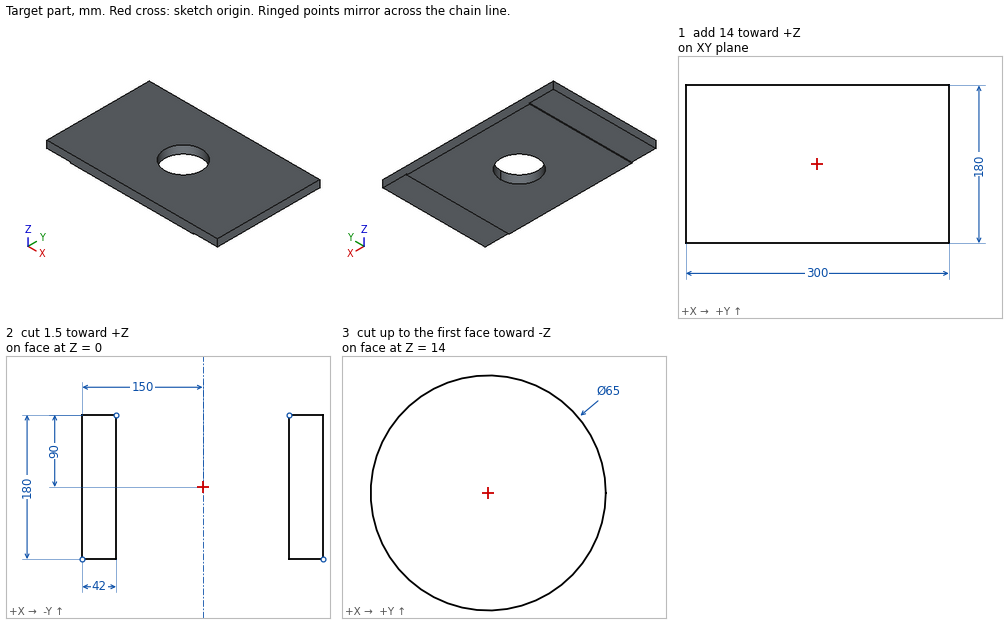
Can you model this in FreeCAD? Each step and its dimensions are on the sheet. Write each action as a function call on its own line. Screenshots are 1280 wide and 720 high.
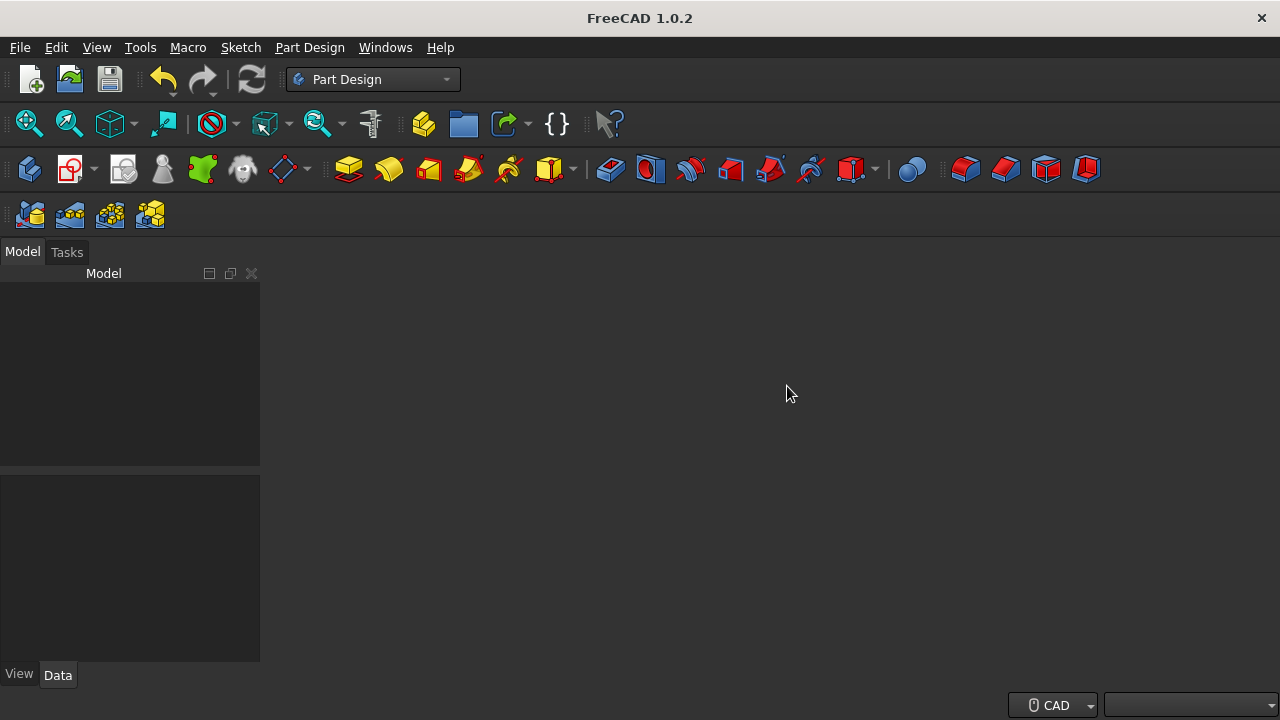
click(30, 80)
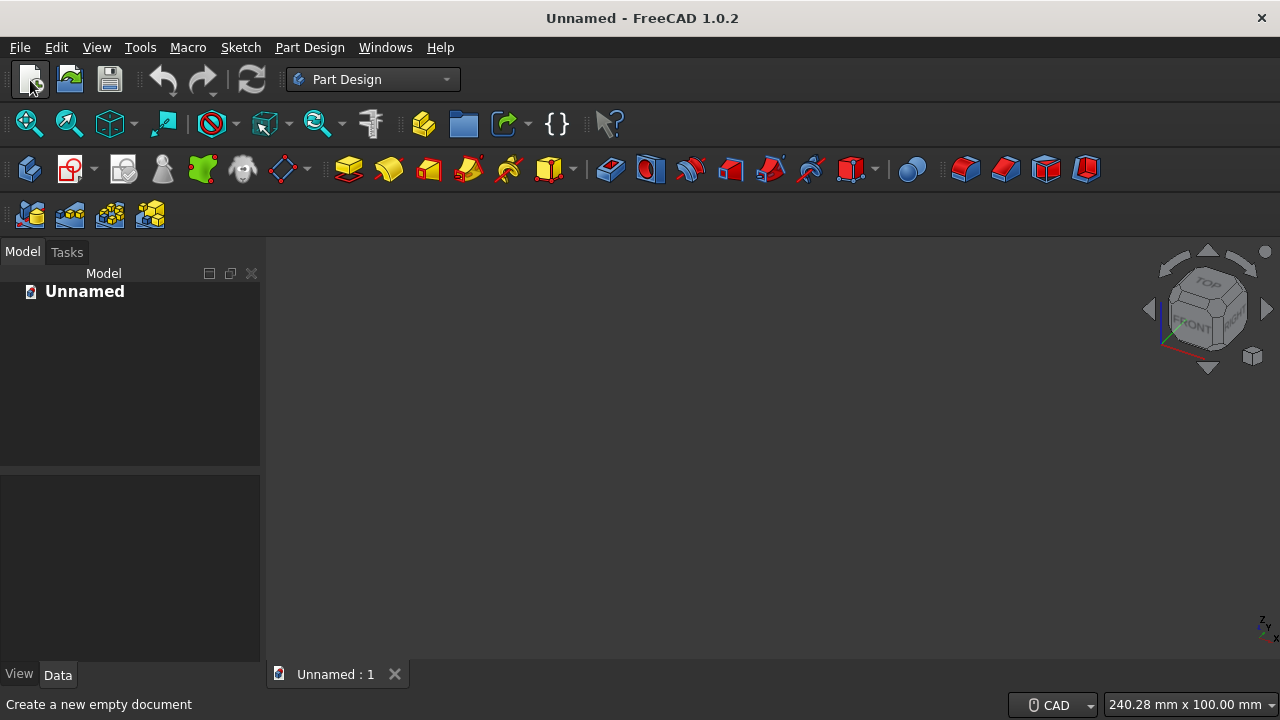
click(70, 170)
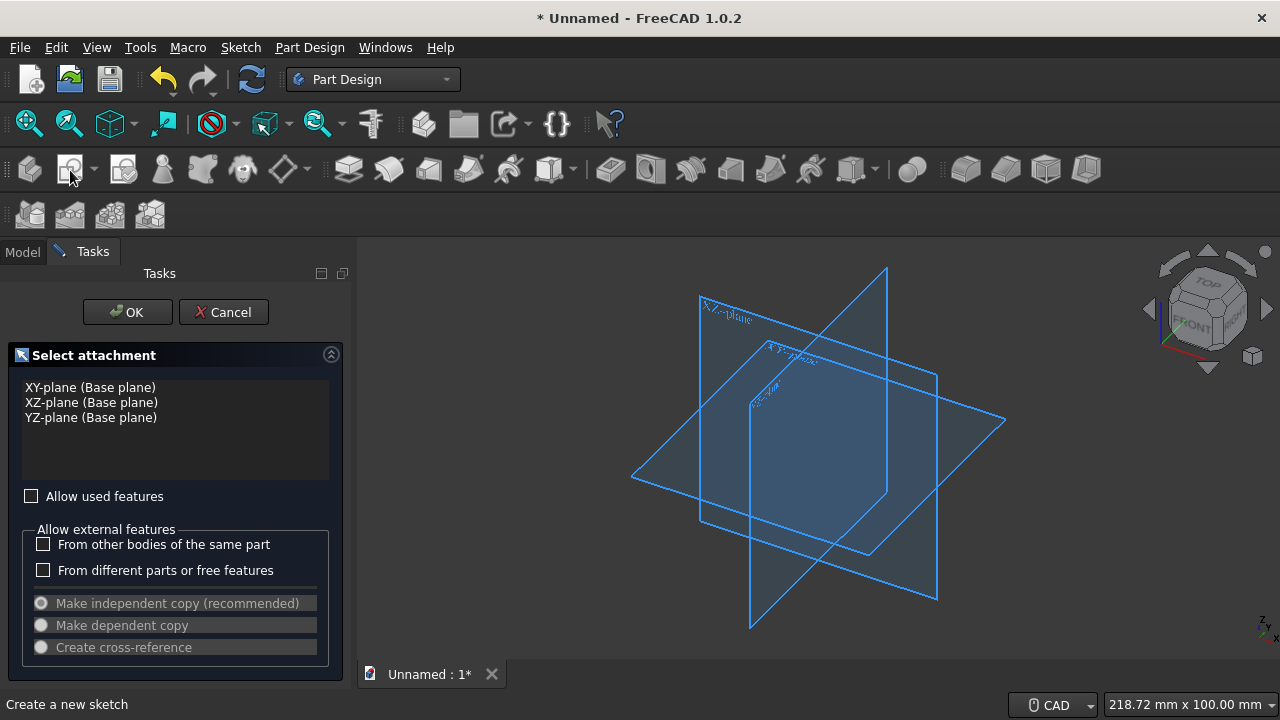
click(82, 388)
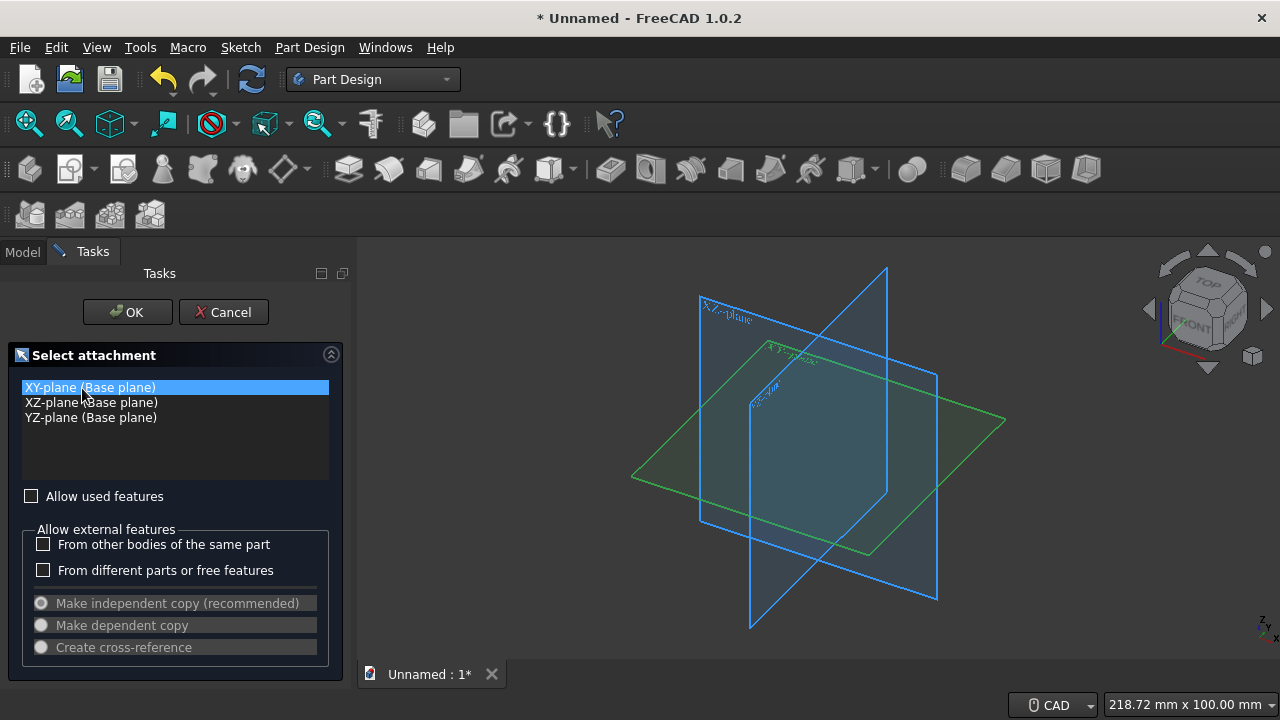
click(128, 312)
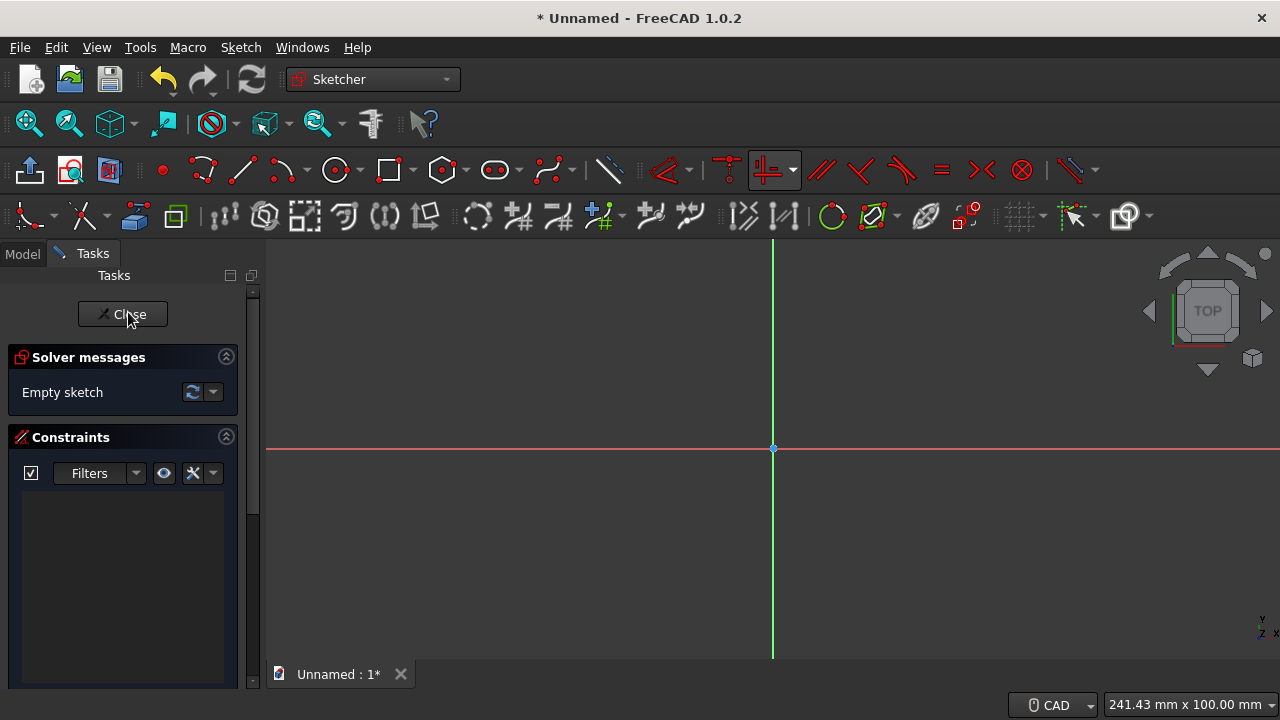
scroll(665, 449, down, 5)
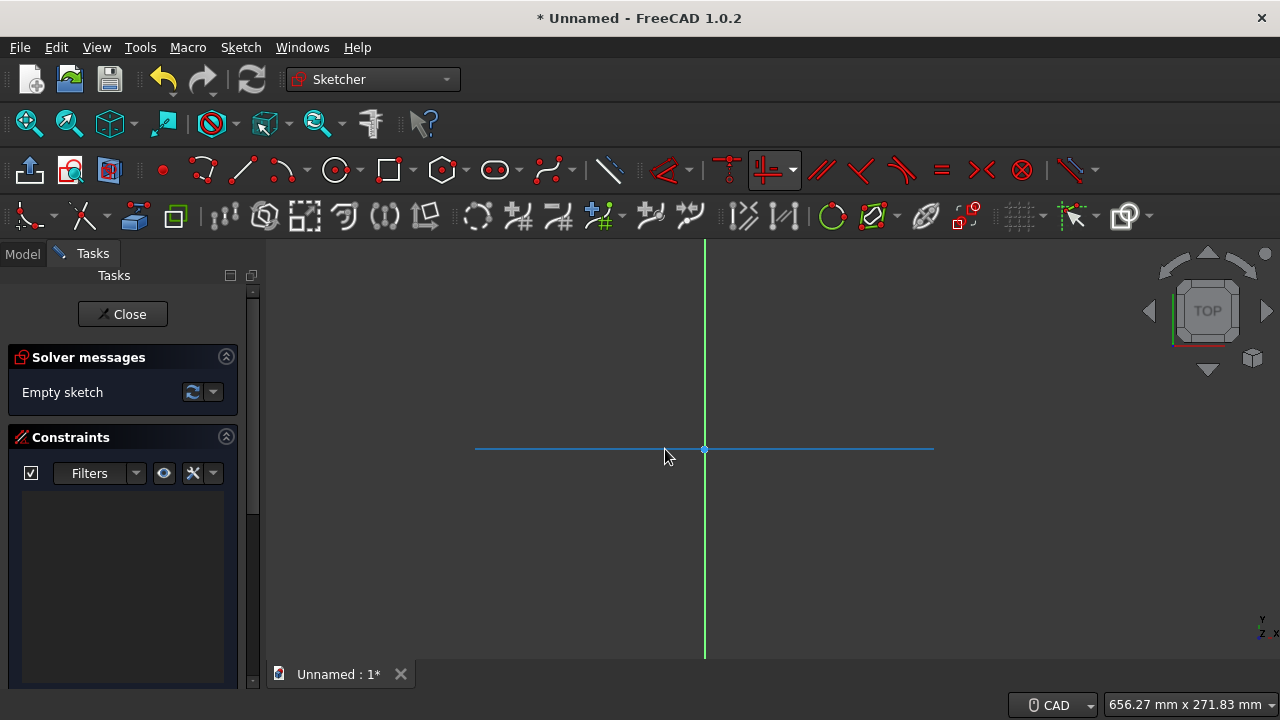
click(416, 170)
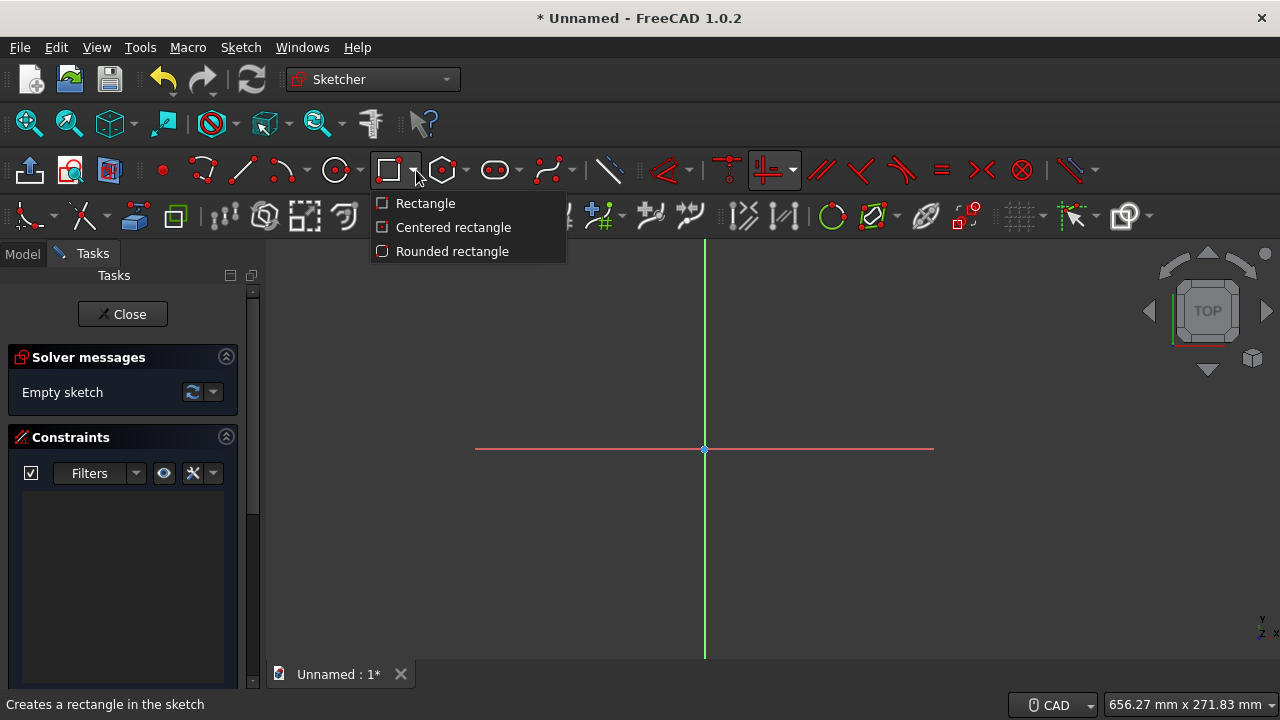
click(468, 227)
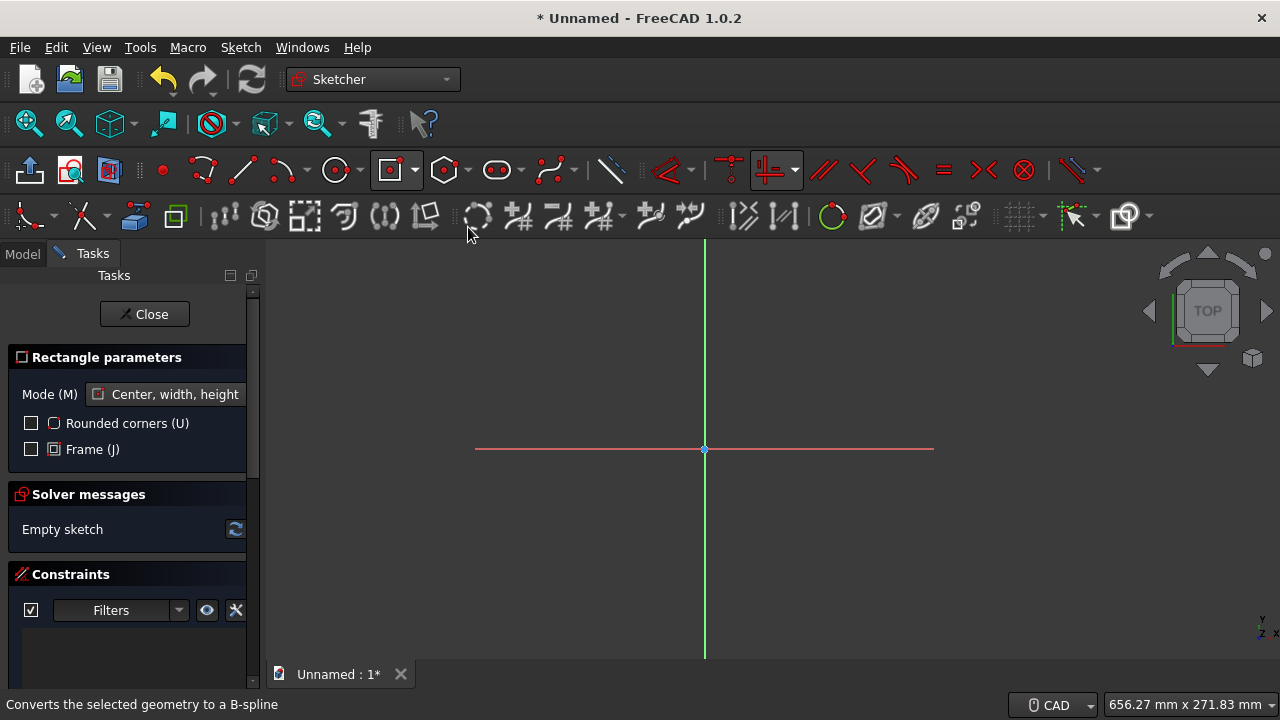
click(705, 449)
click(937, 310)
key(Escape)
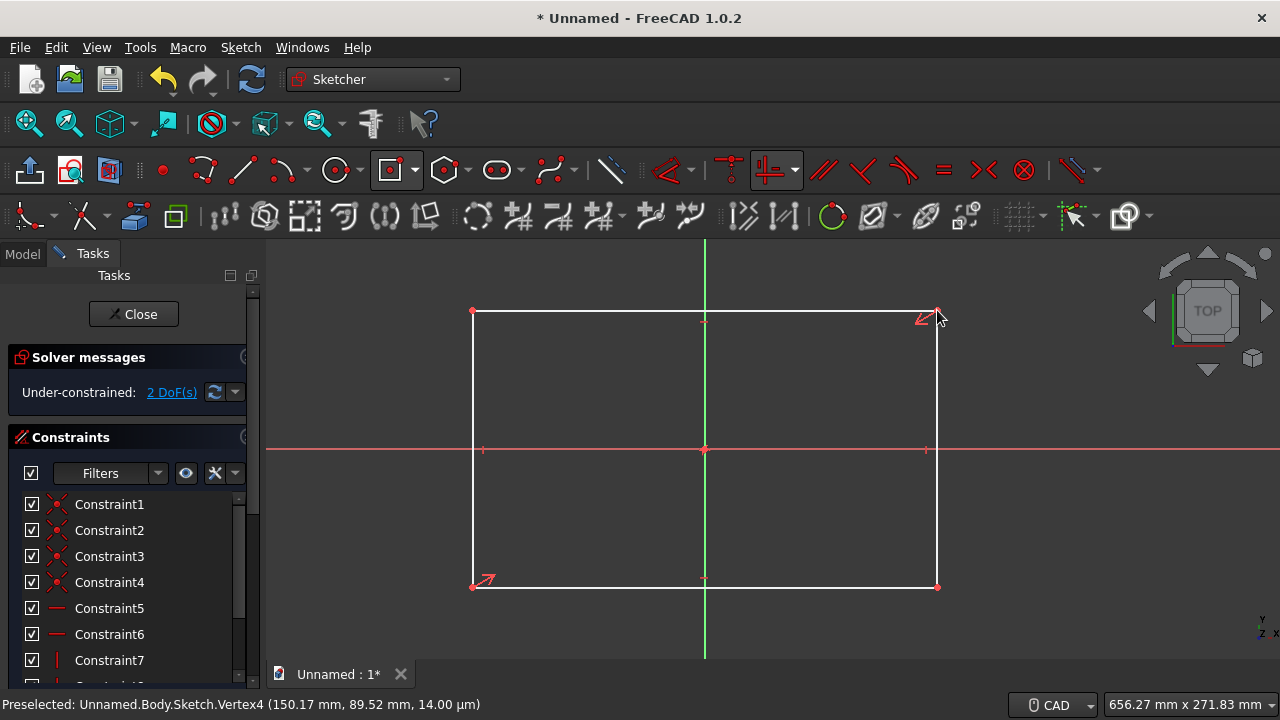
click(666, 170)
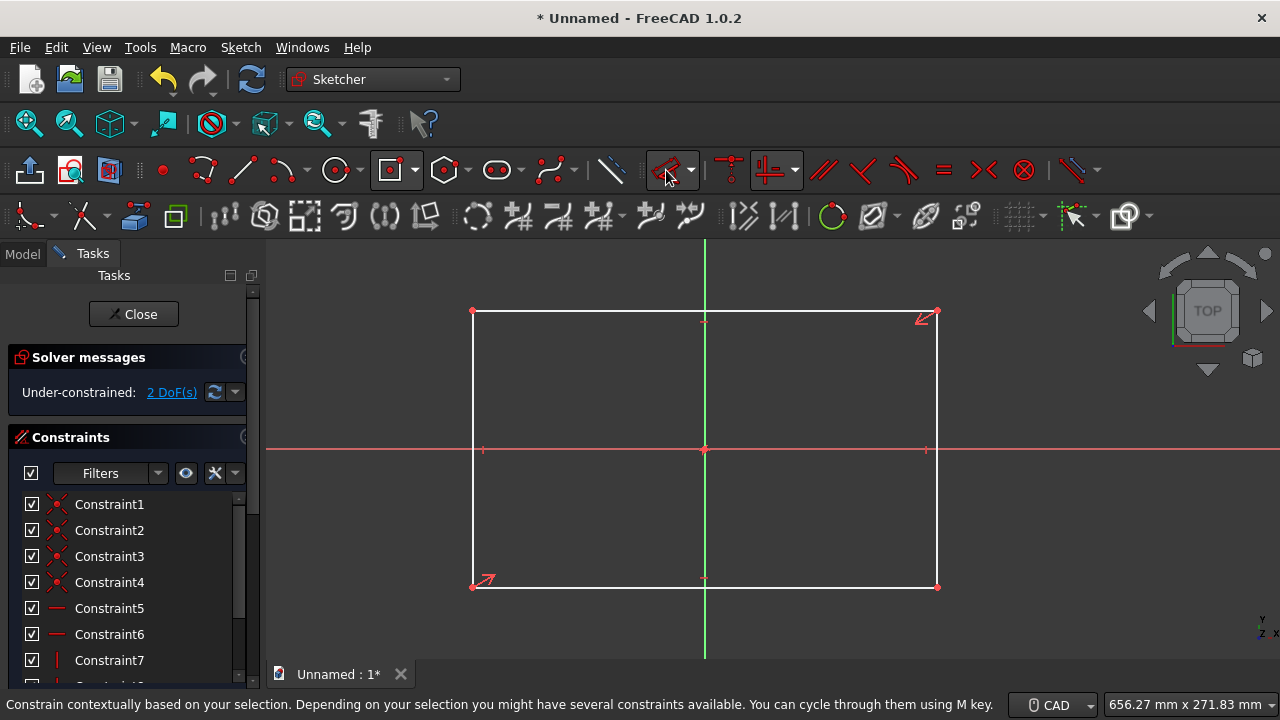
click(612, 588)
click(598, 622)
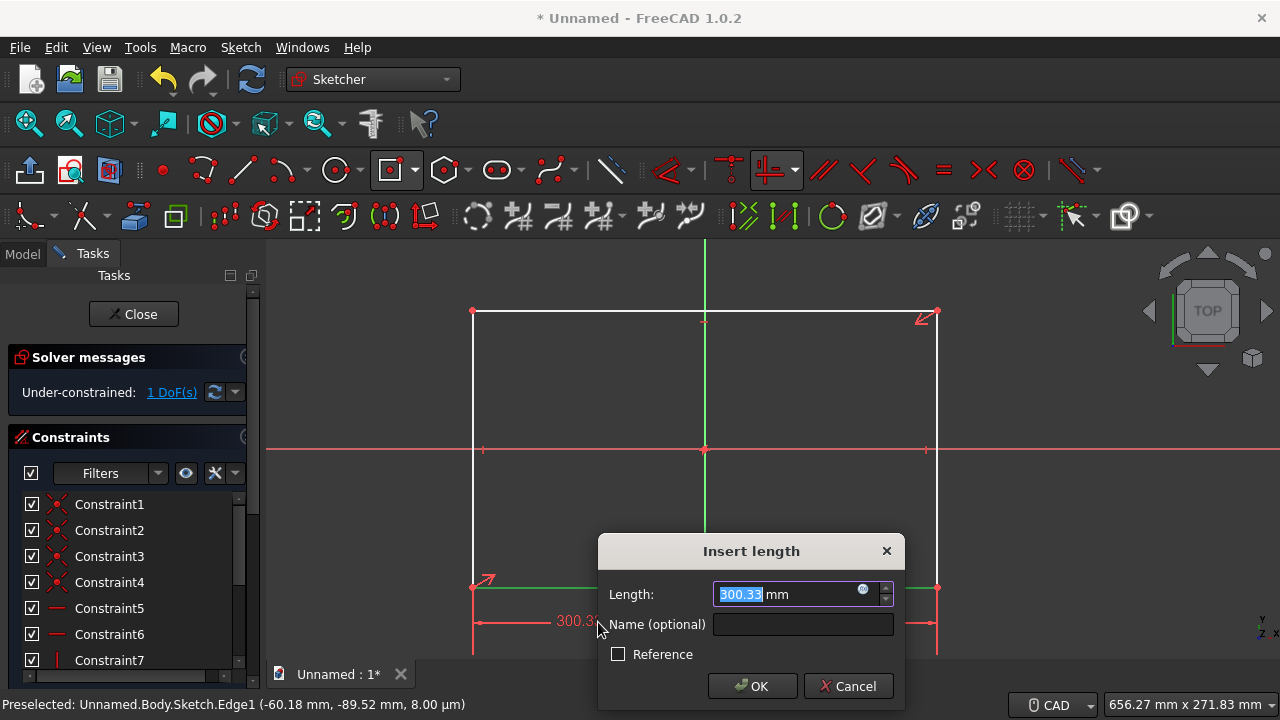
text(300)
key(Return)